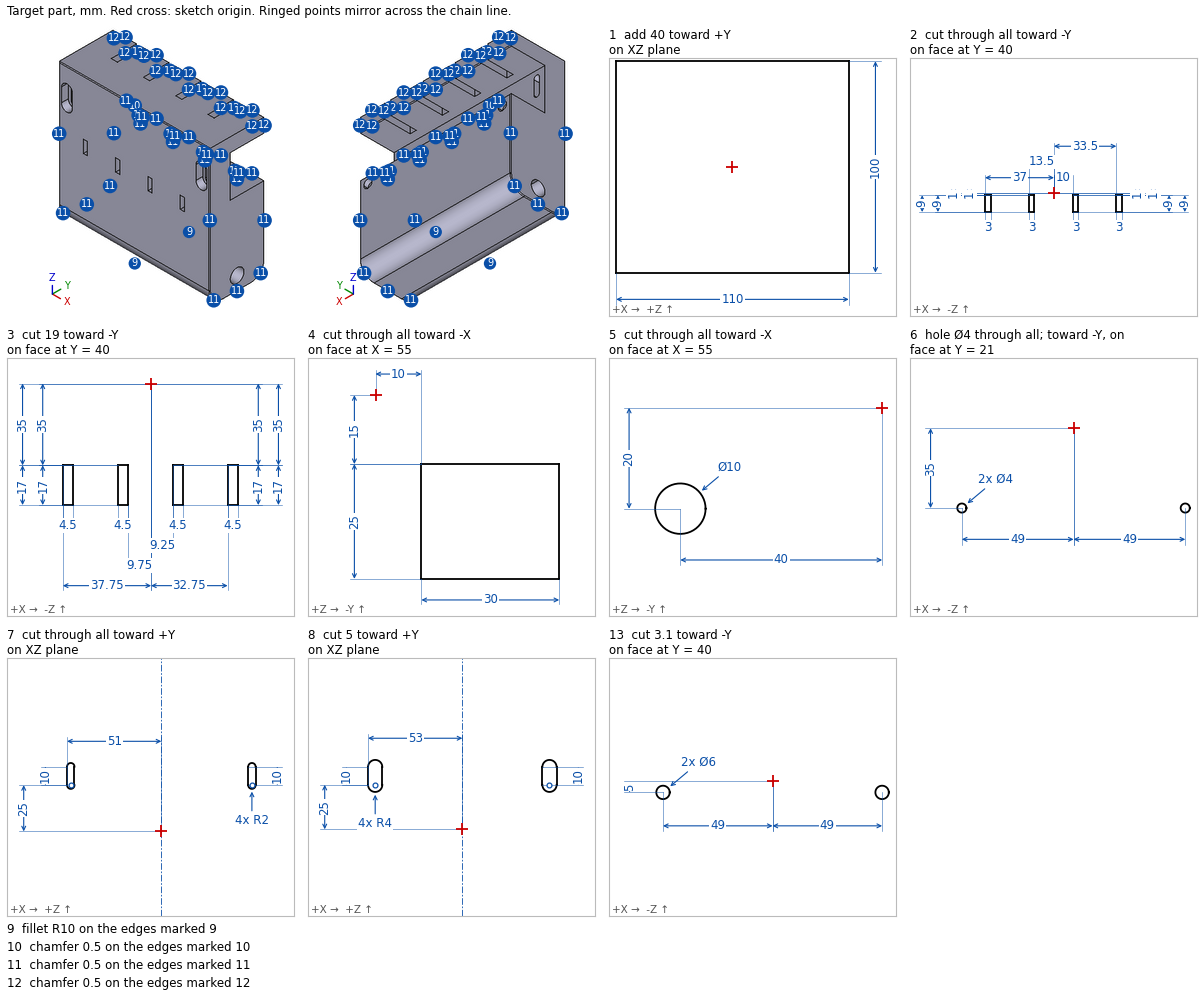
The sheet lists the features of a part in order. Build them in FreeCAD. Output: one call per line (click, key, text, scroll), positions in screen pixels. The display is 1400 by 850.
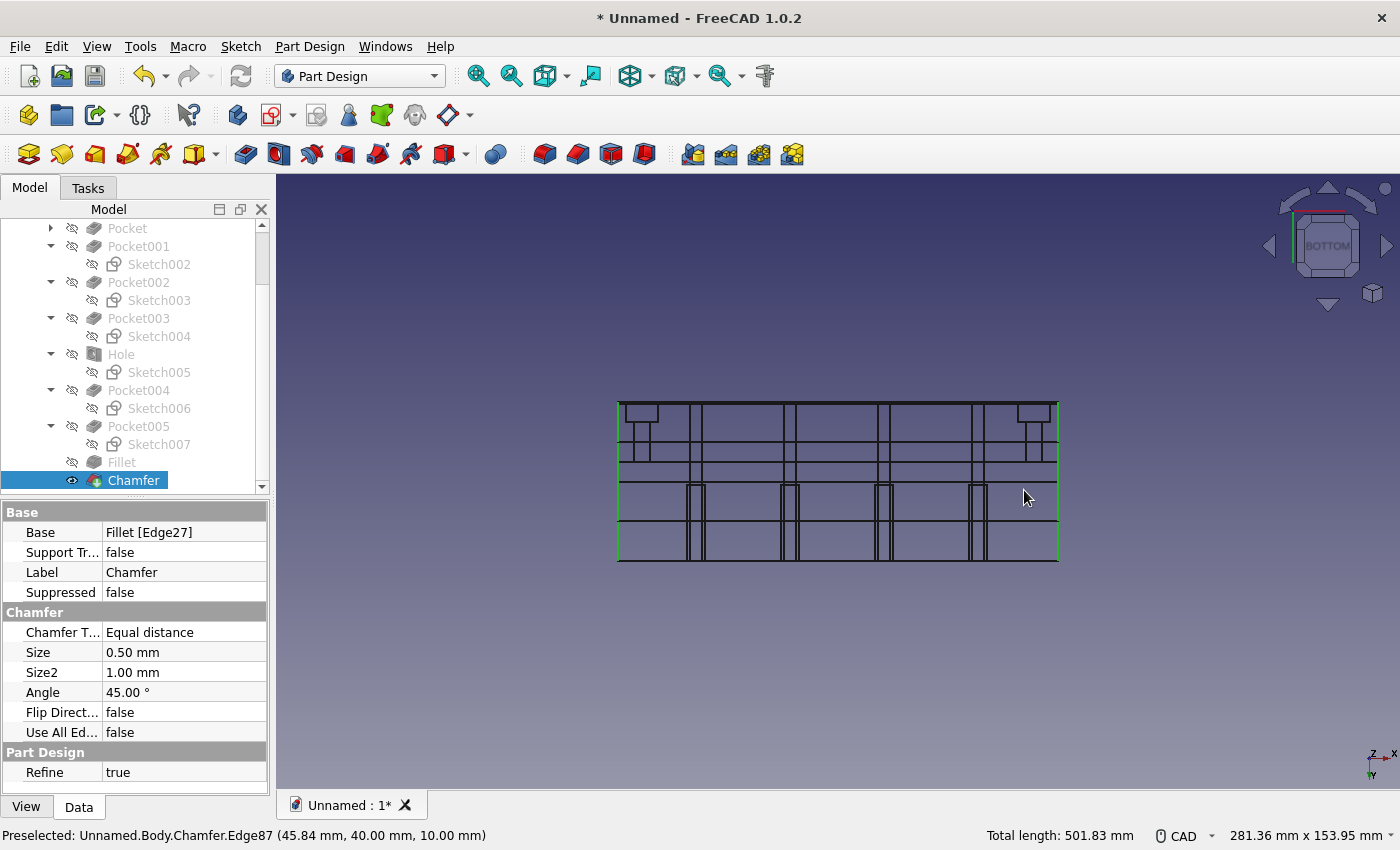
key(4)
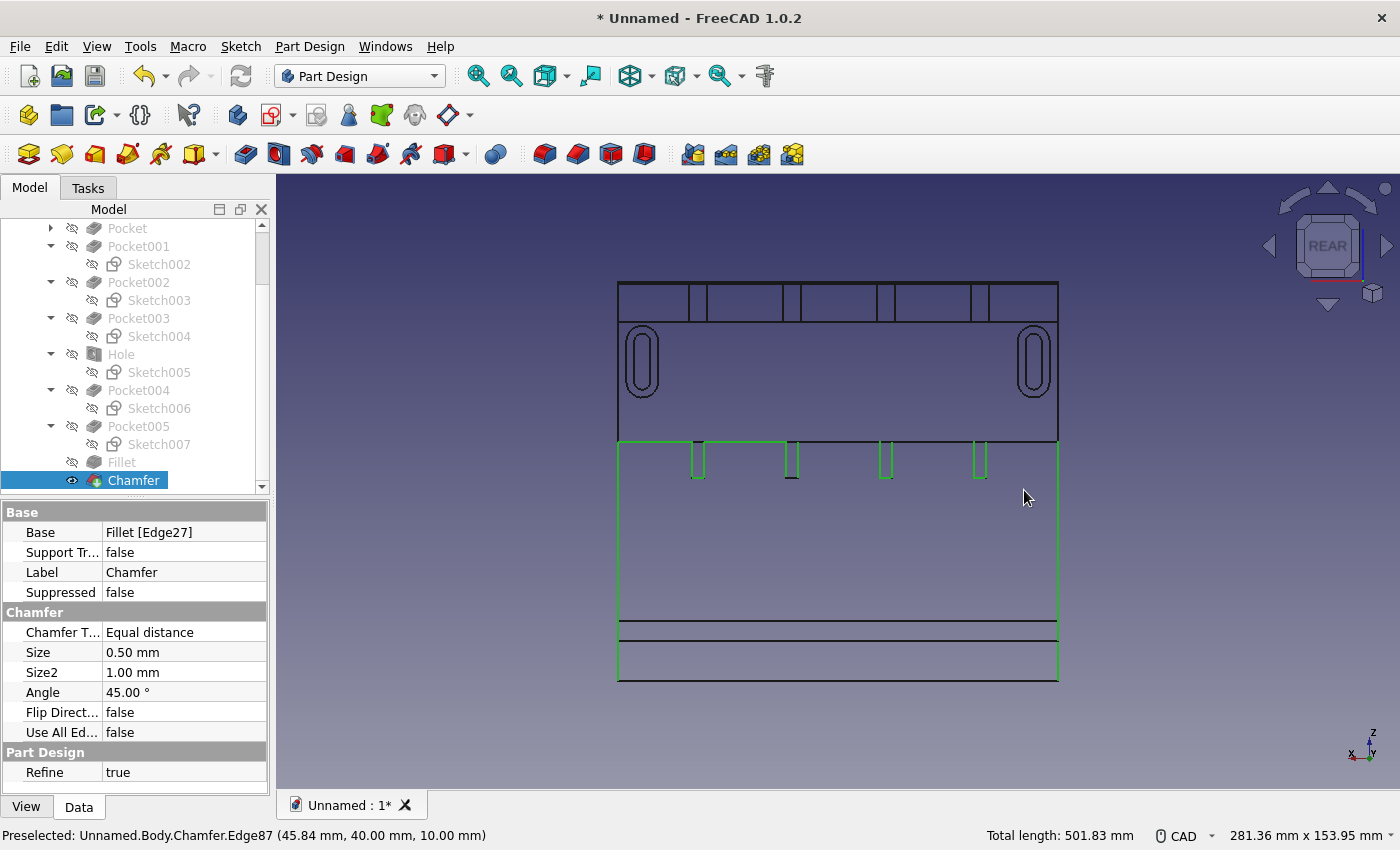
click(1022, 441, ctrl)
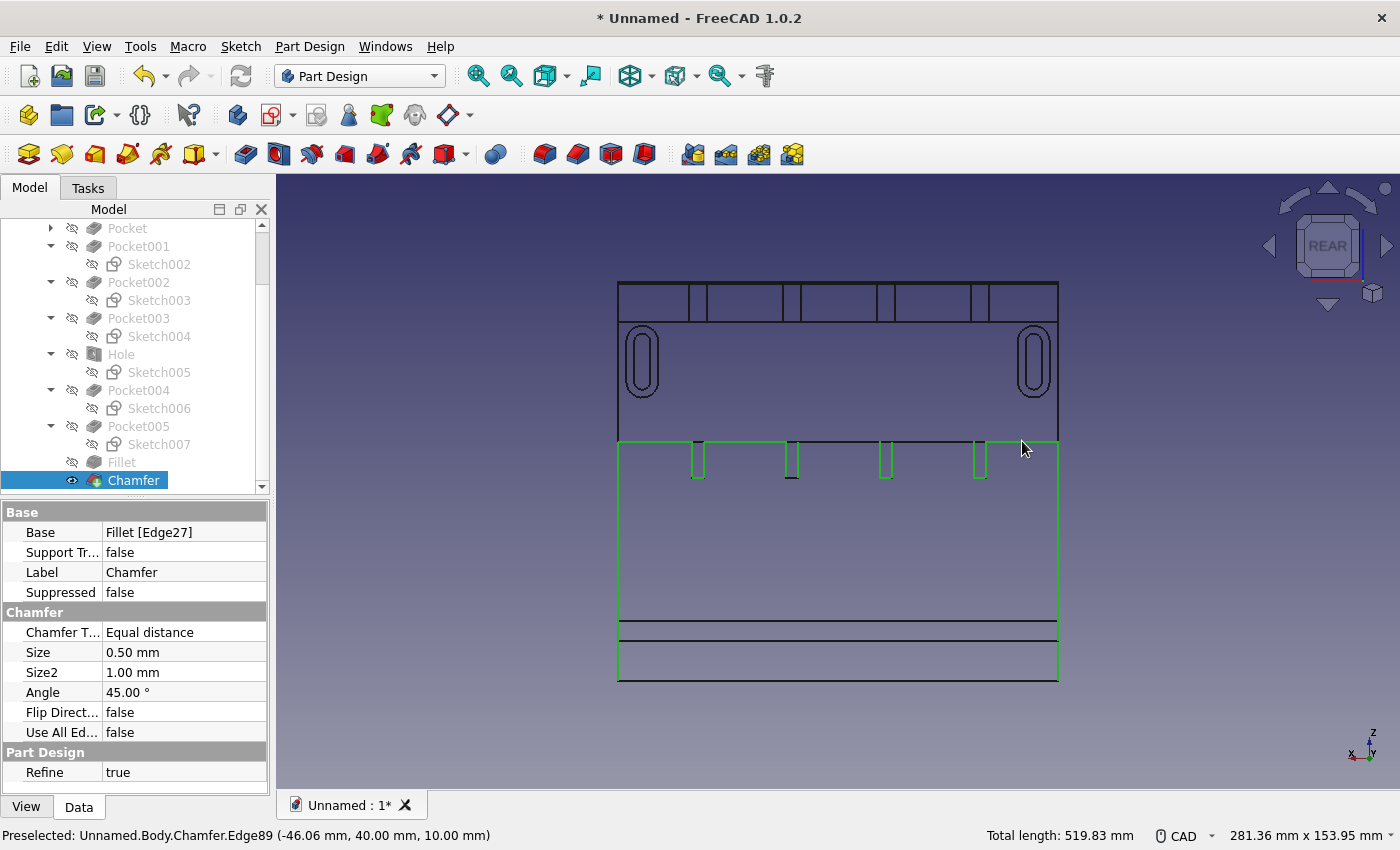
click(933, 441, ctrl)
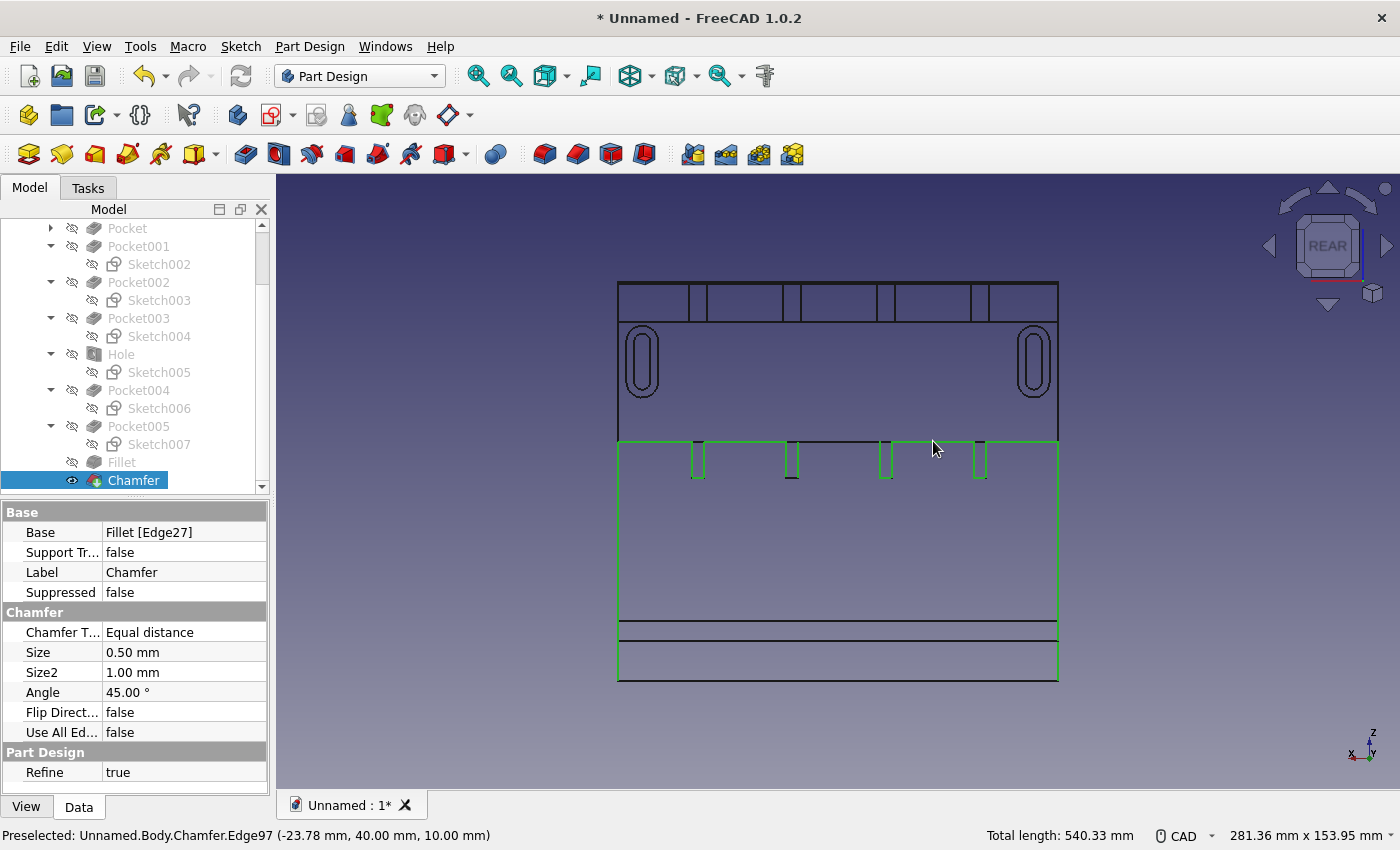
click(839, 441, ctrl)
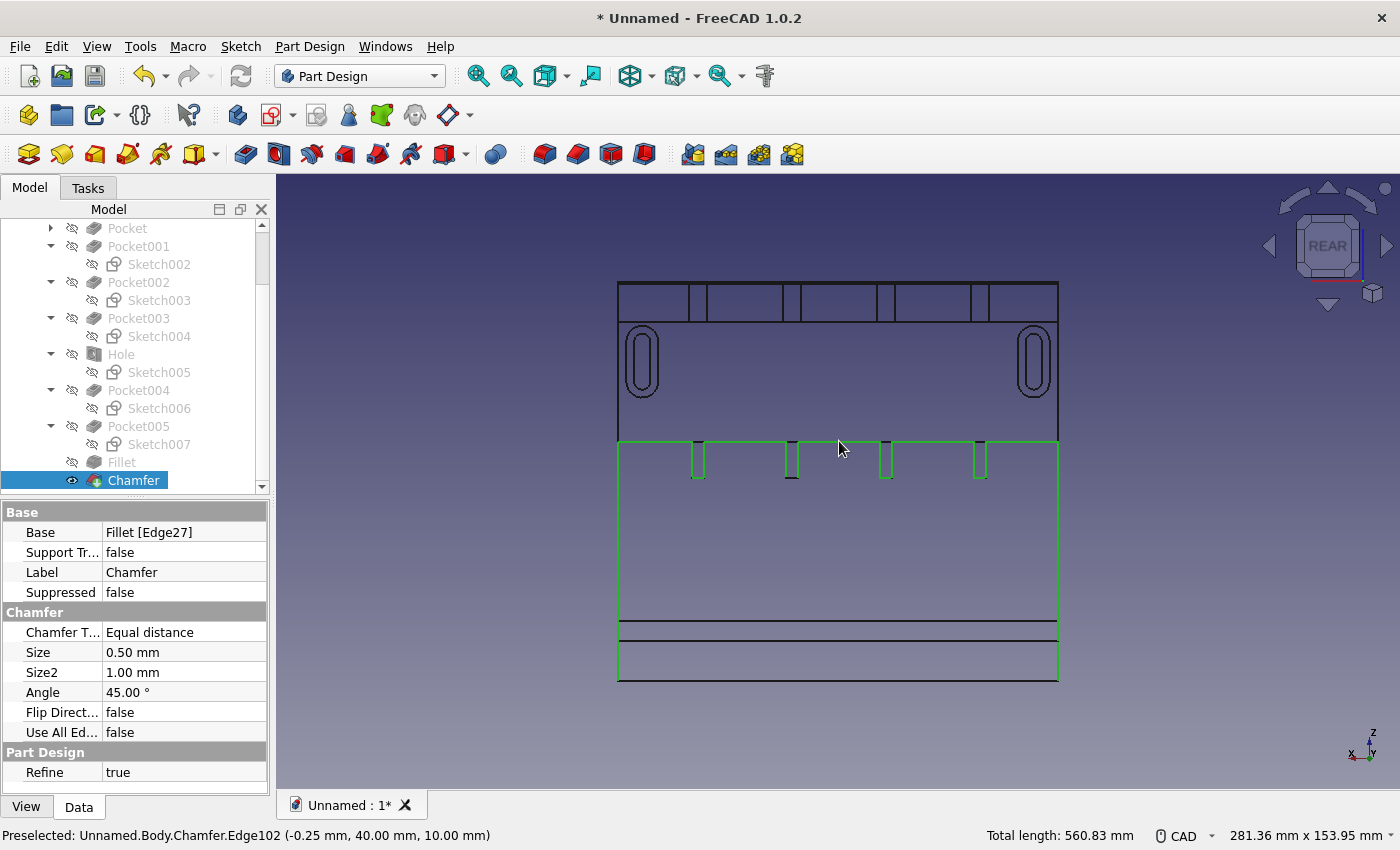
click(792, 477, ctrl)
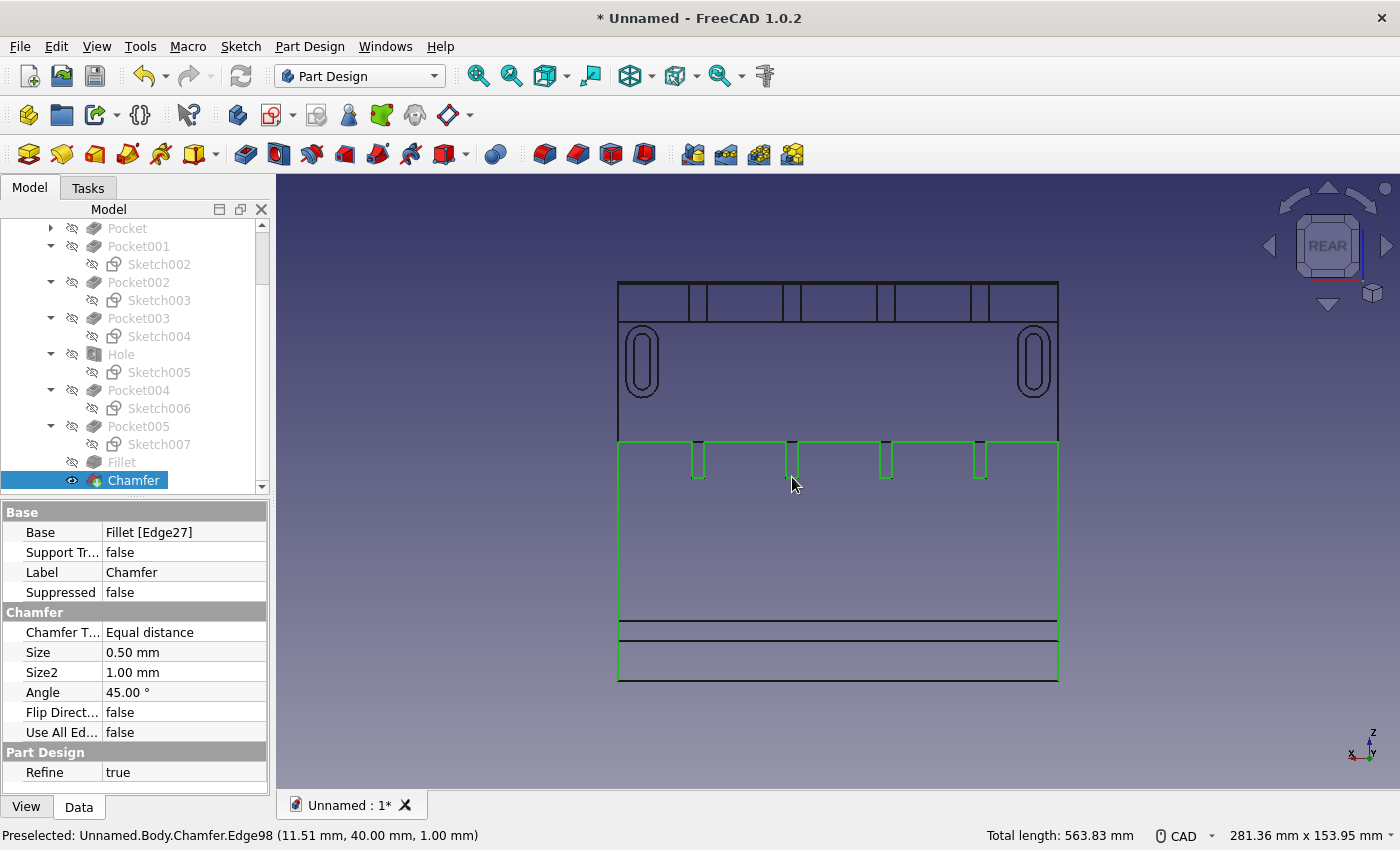
key(v)
key(1)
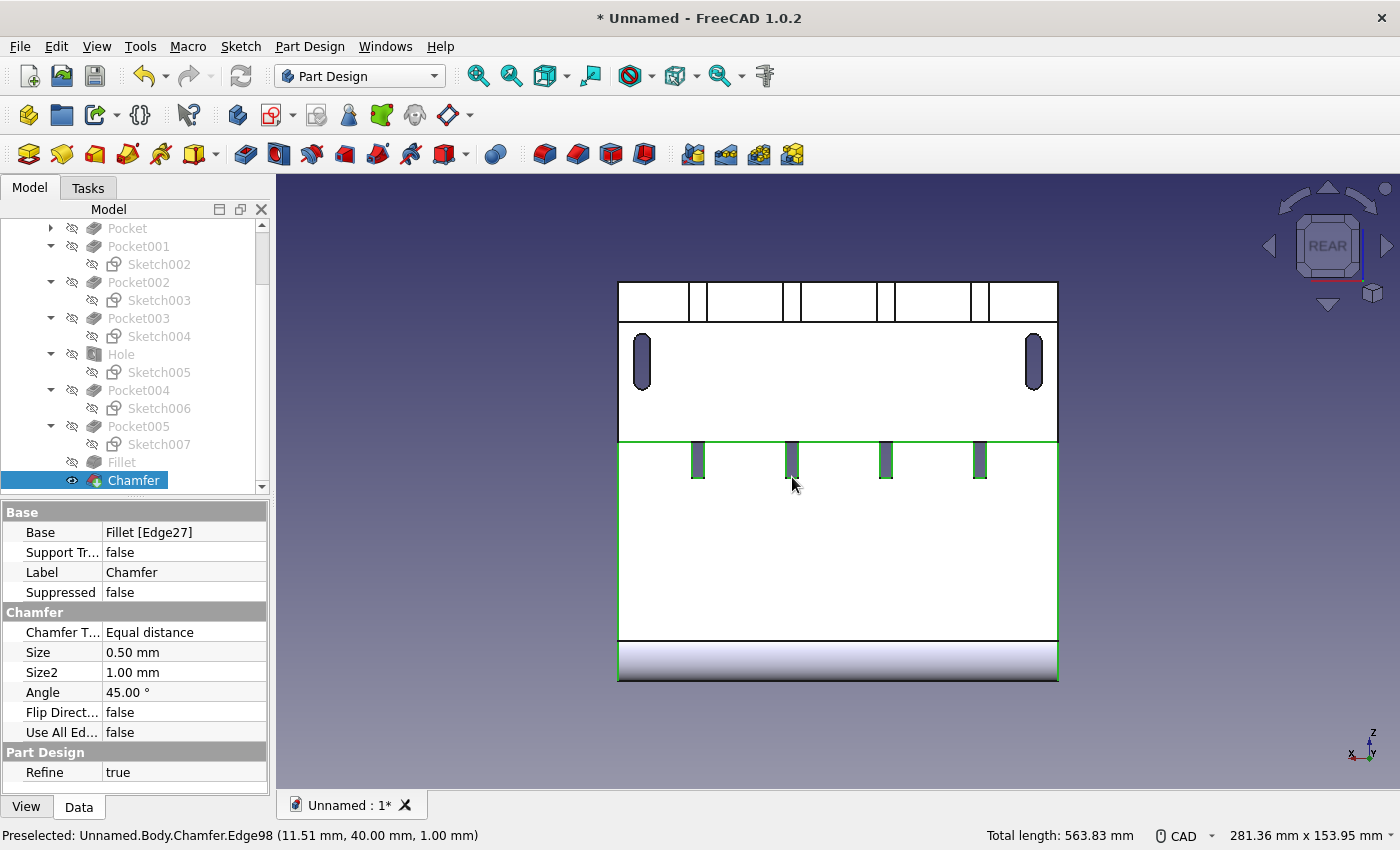
click(578, 154)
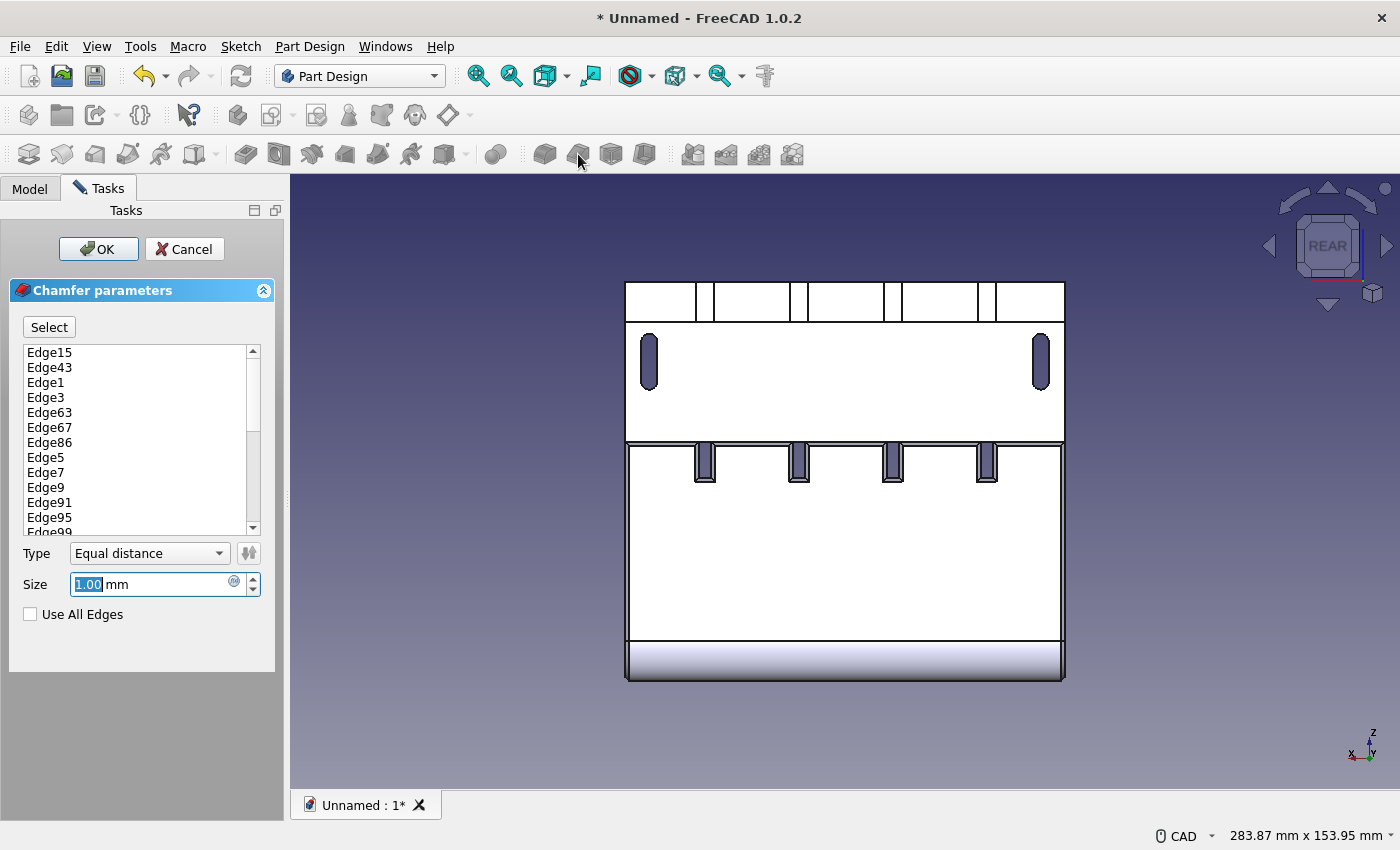
text(0.5)
key(Tab)